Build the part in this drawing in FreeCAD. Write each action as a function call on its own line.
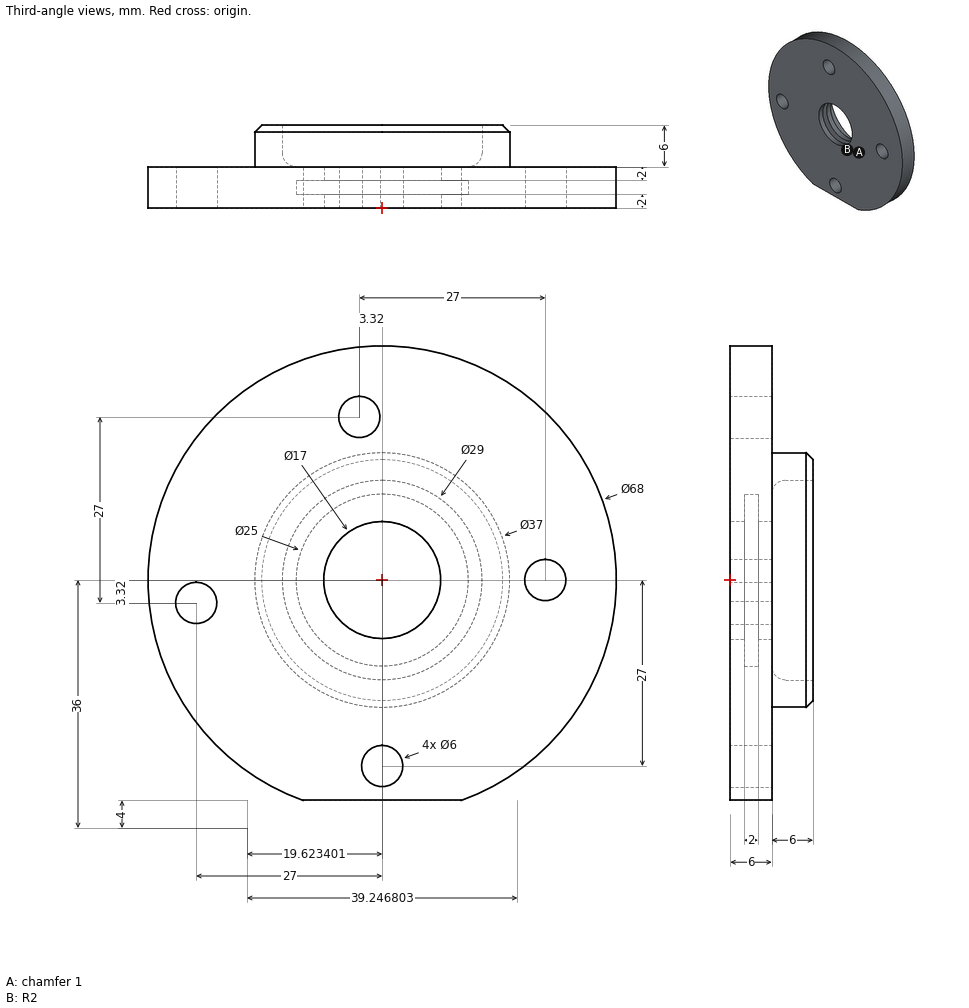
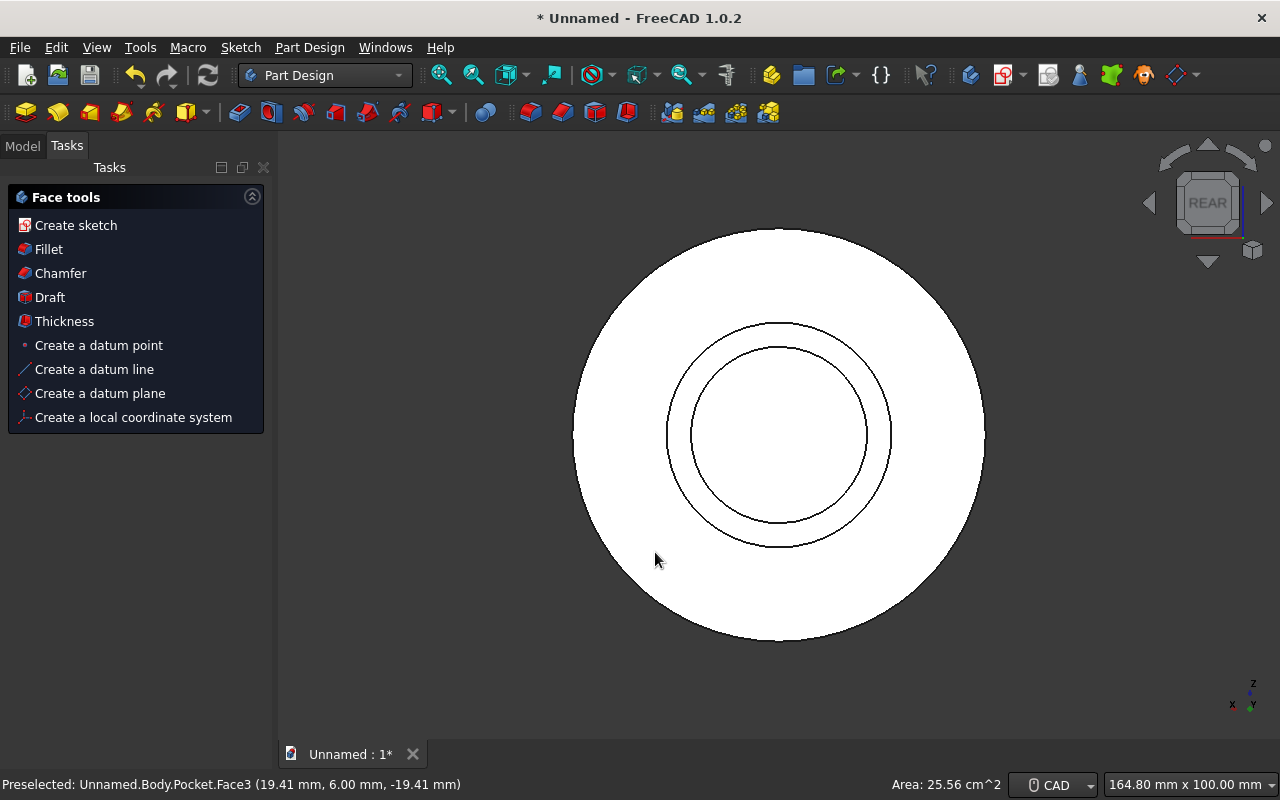
click(1004, 76)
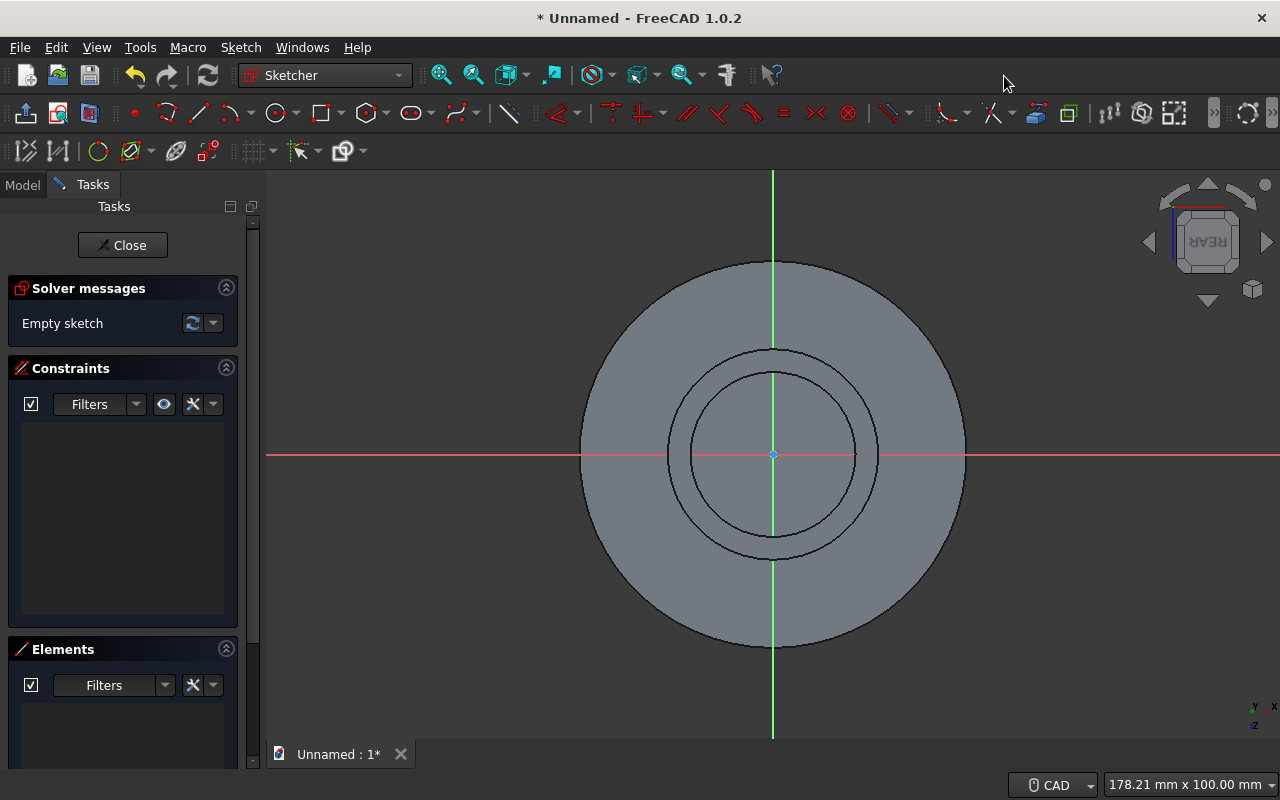
scroll(795, 454, up, 7)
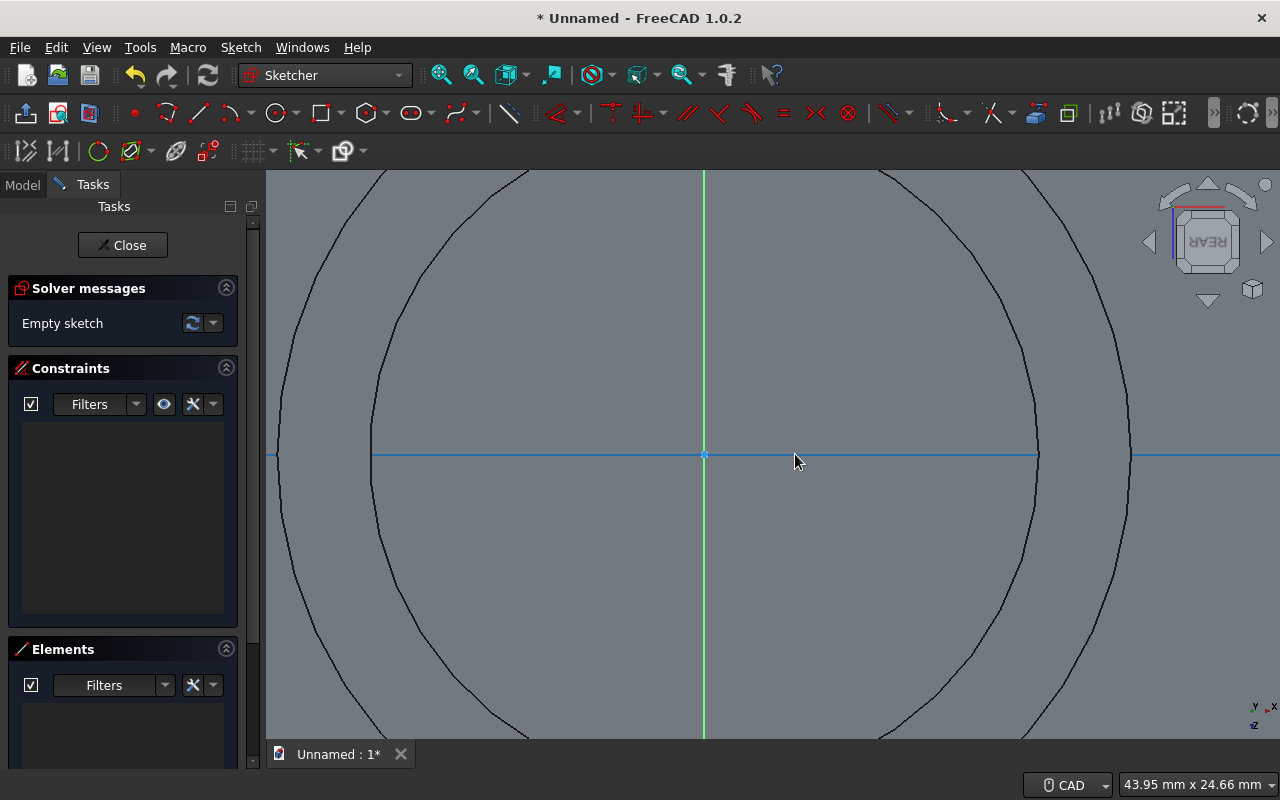
click(276, 114)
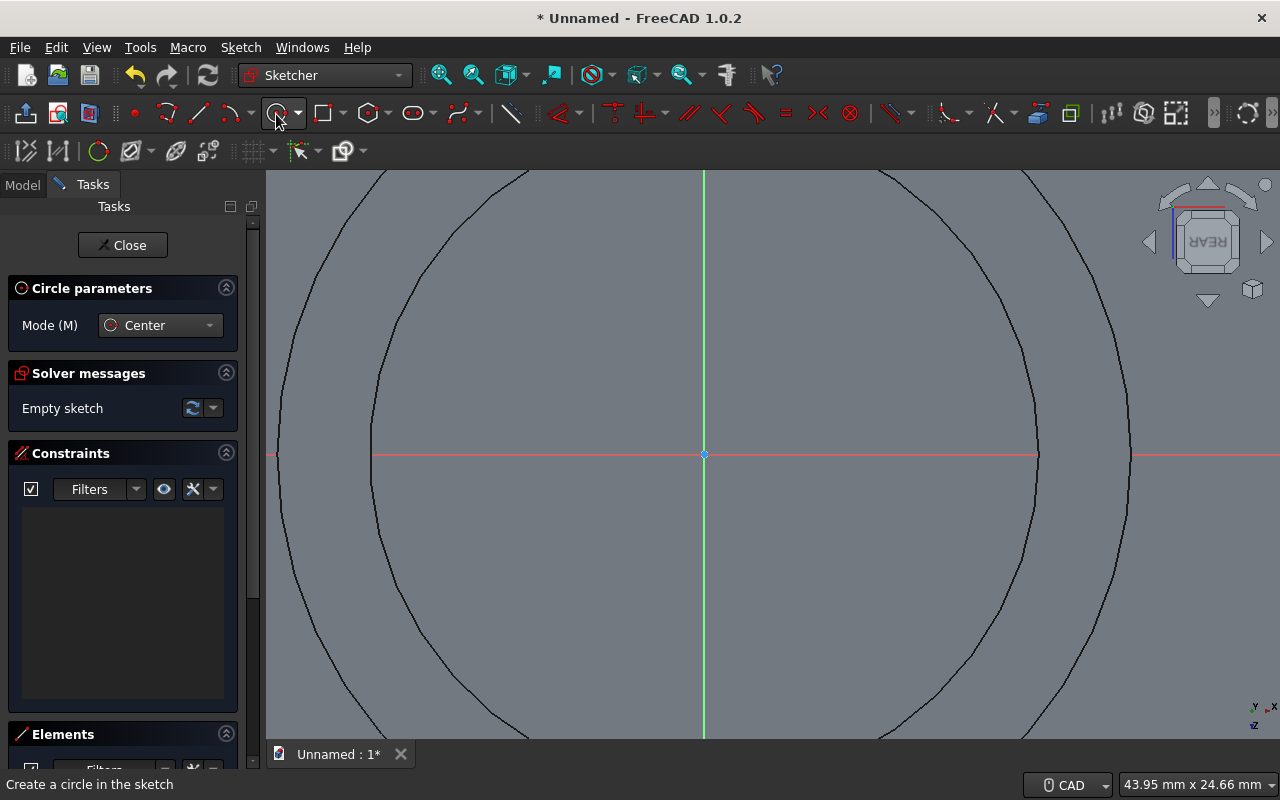
click(704, 454)
click(843, 316)
key(Escape)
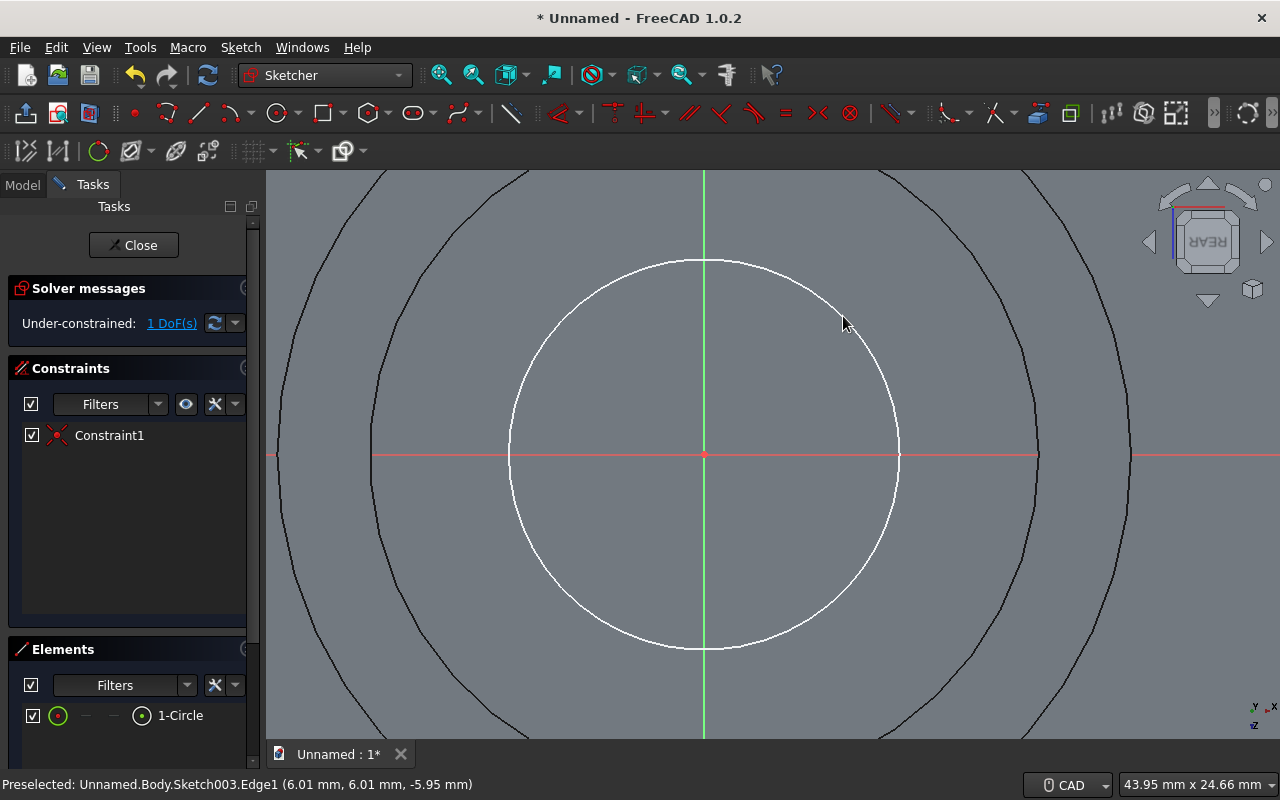
click(558, 114)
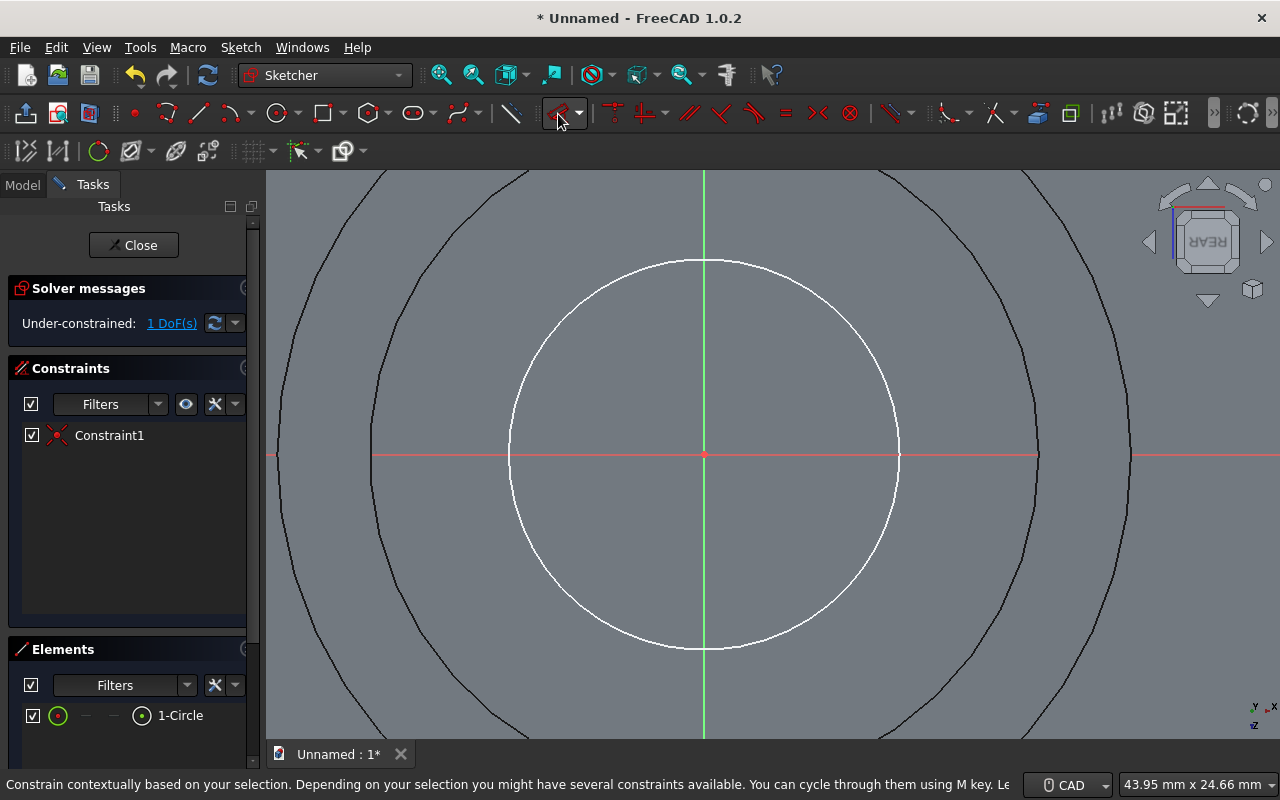
click(842, 316)
click(865, 293)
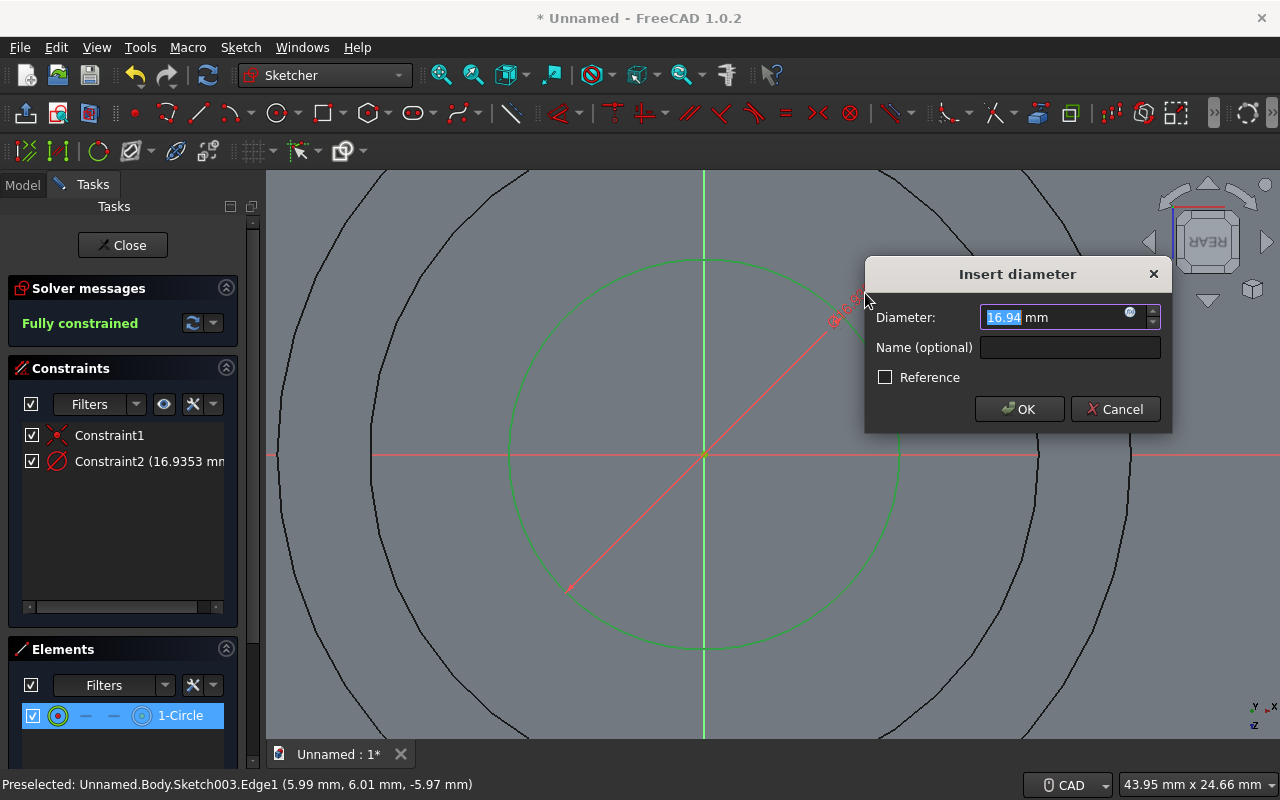
text(17)
key(Return)
key(Escape)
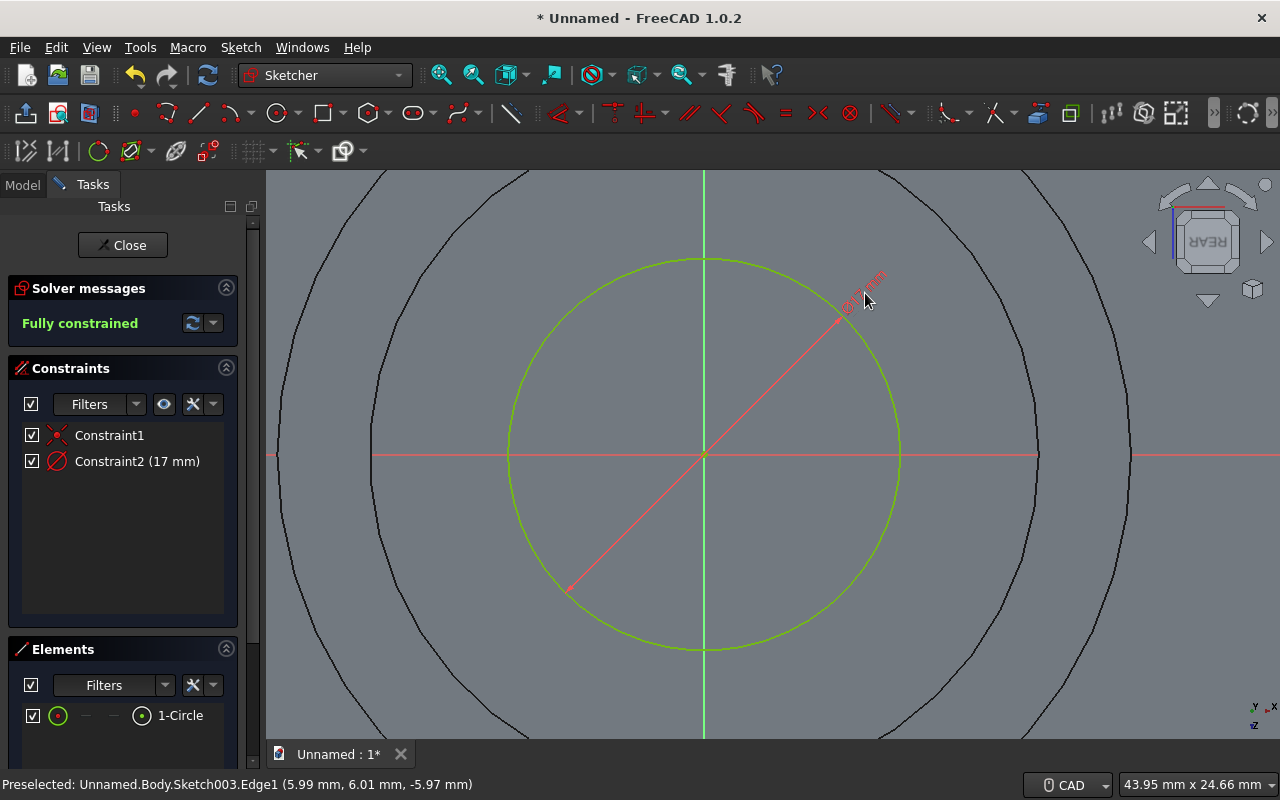
click(123, 245)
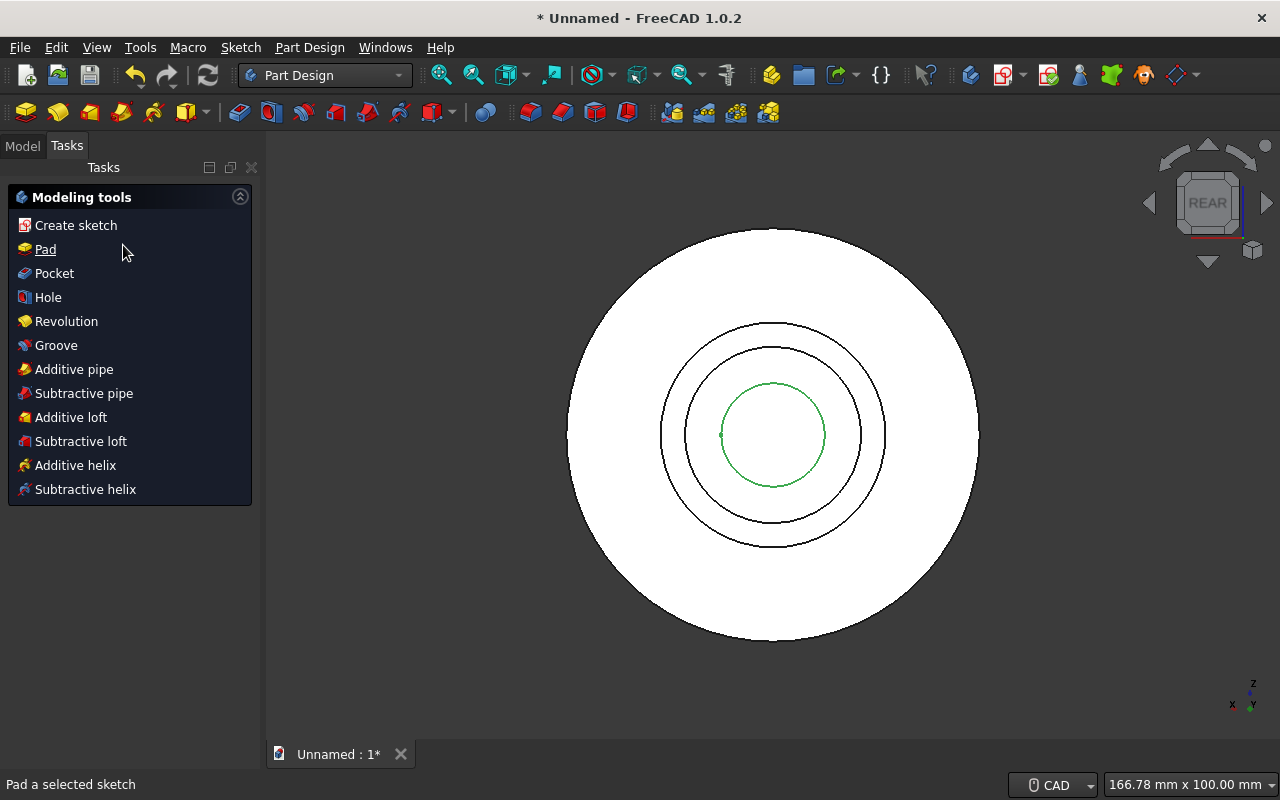
click(240, 112)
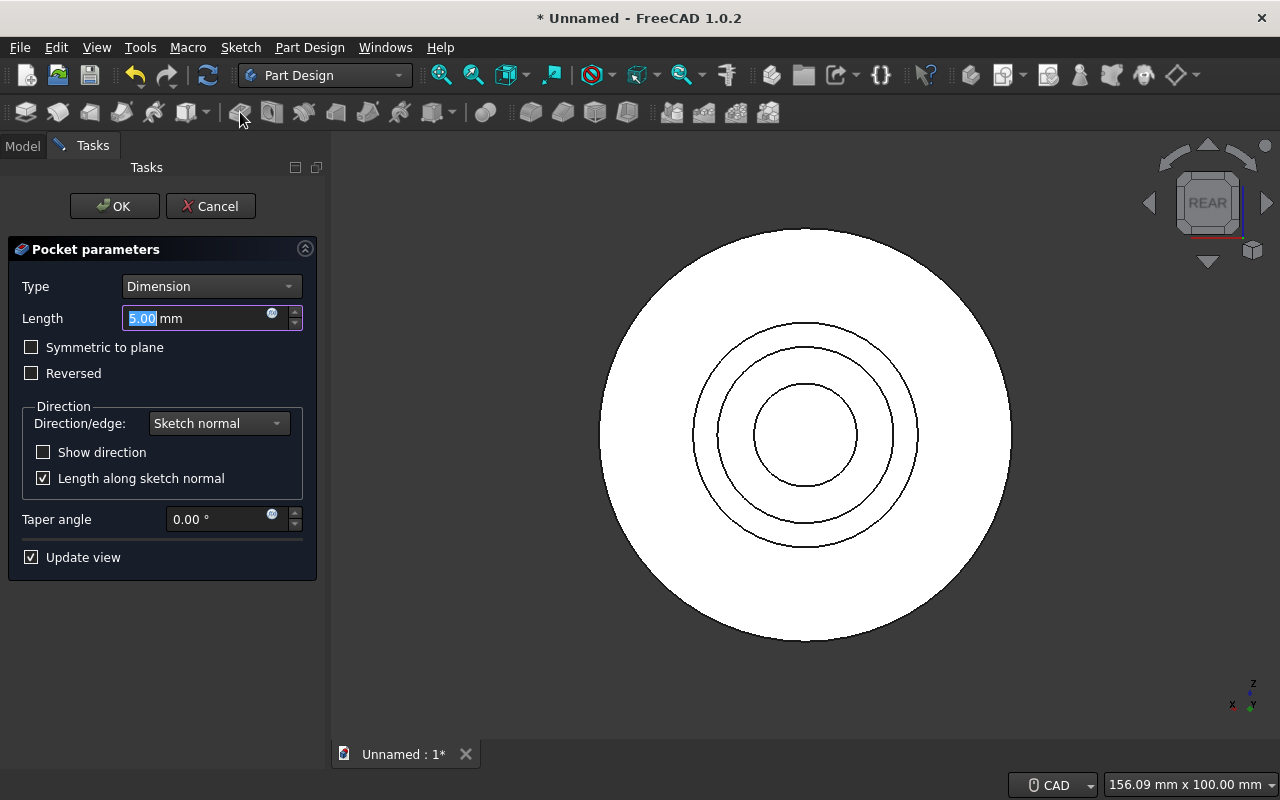
text(2)
key(Tab)